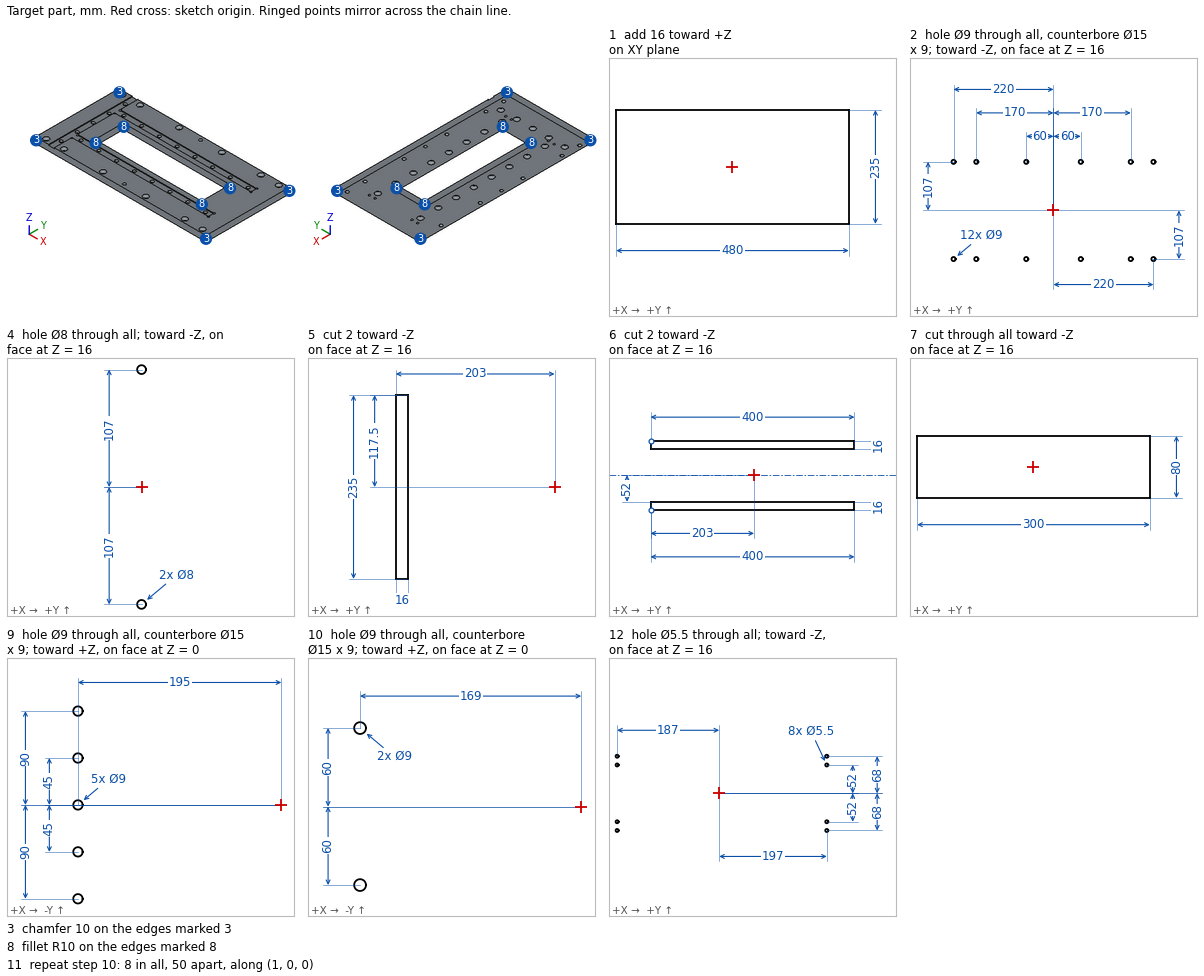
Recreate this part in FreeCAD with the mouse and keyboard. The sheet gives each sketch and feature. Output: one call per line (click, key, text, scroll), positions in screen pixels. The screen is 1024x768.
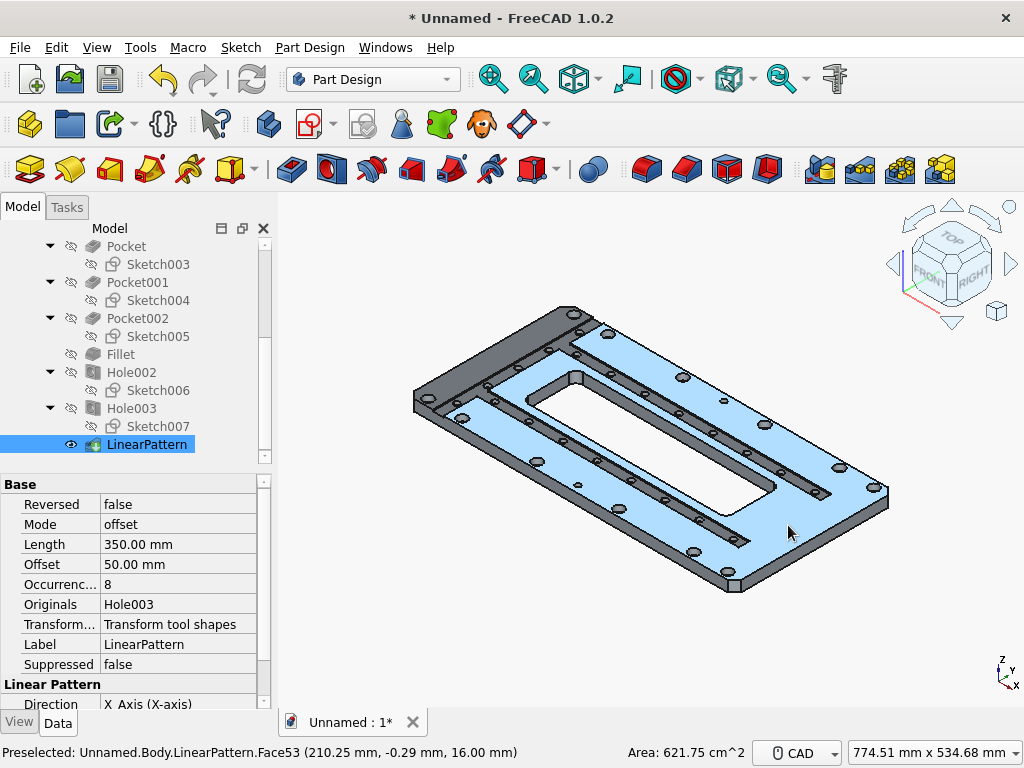
click(310, 124)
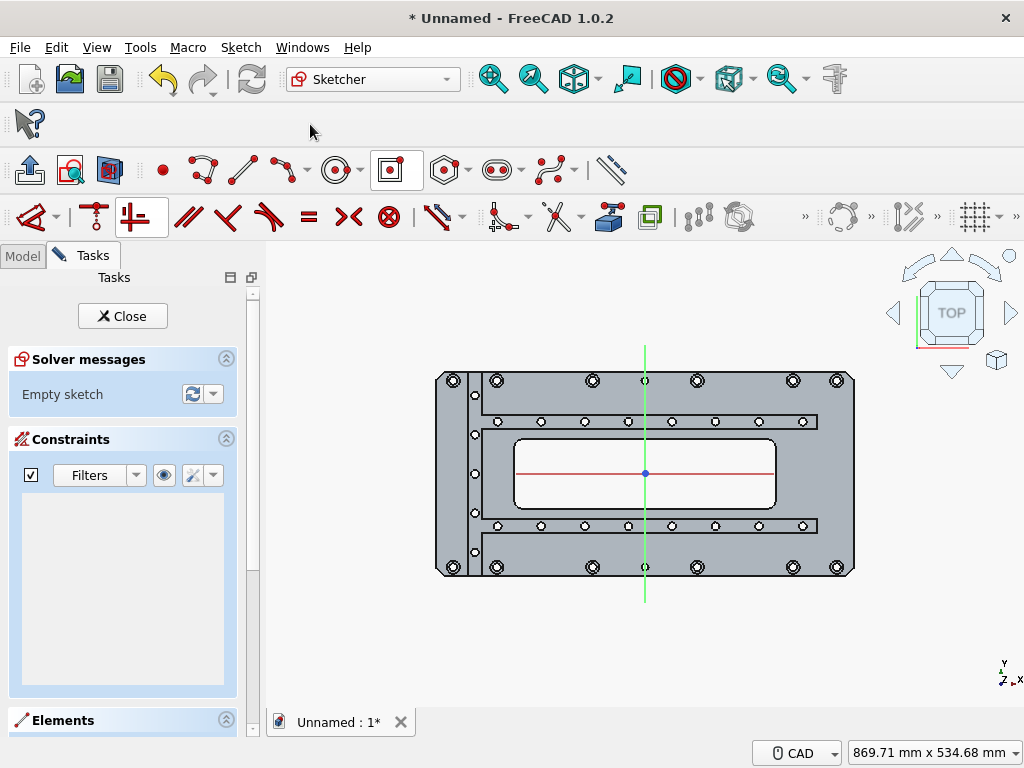
click(336, 170)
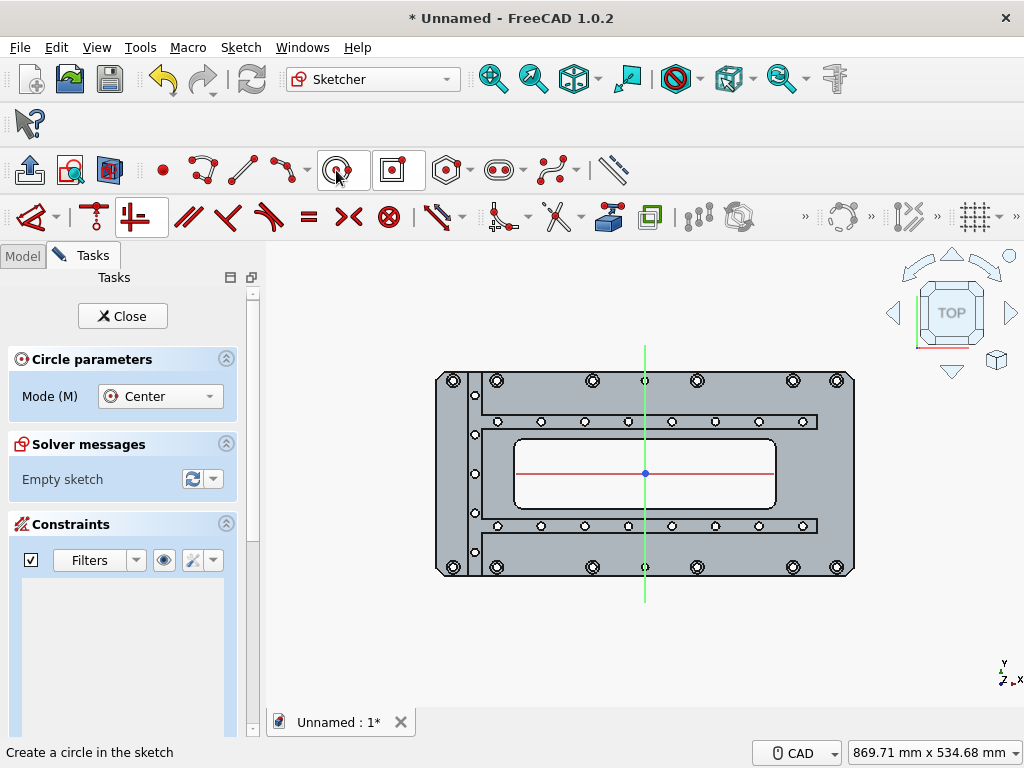
scroll(817, 533, up, 12)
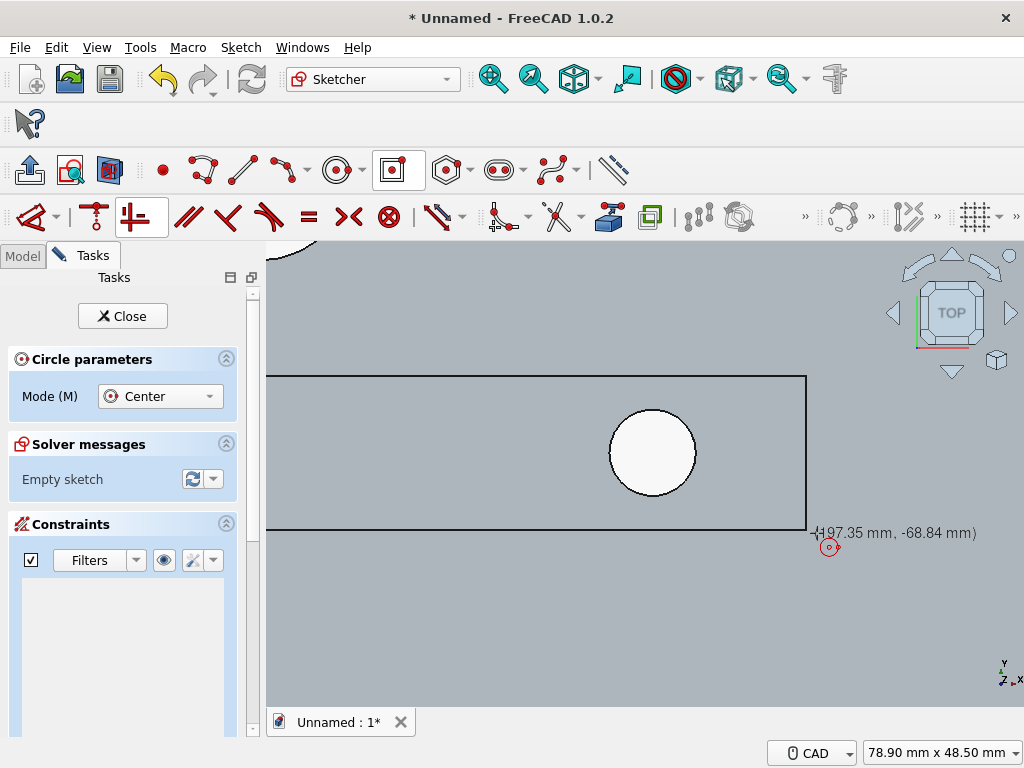
scroll(778, 548, down, 11)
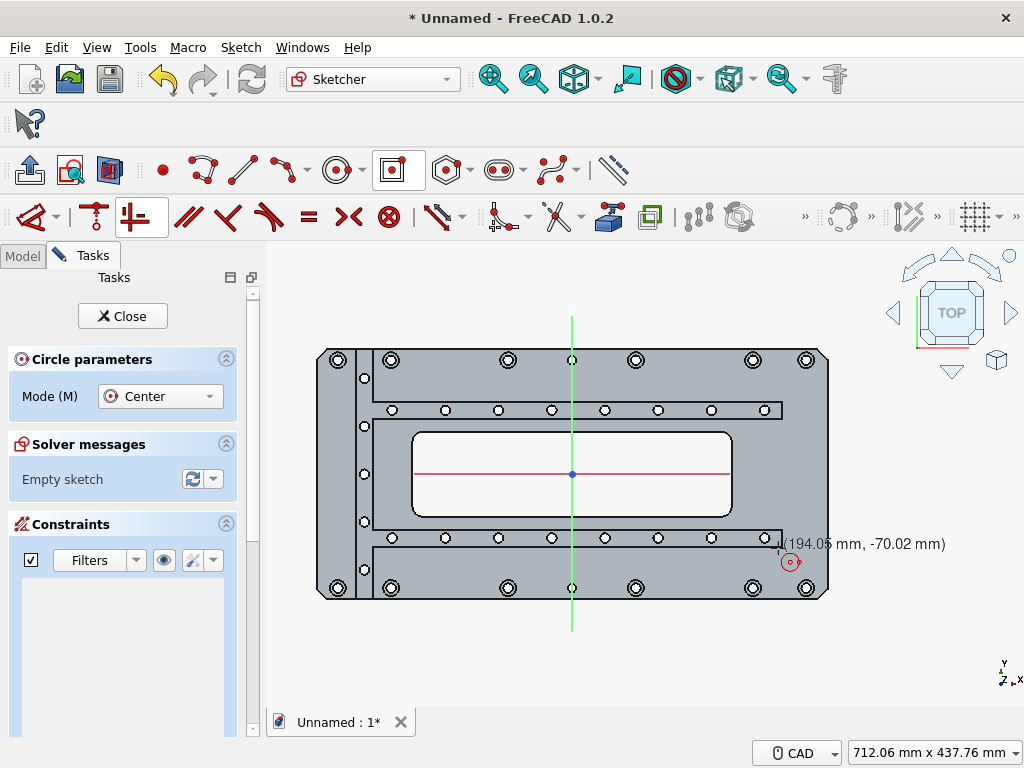
click(782, 547)
move(784, 544)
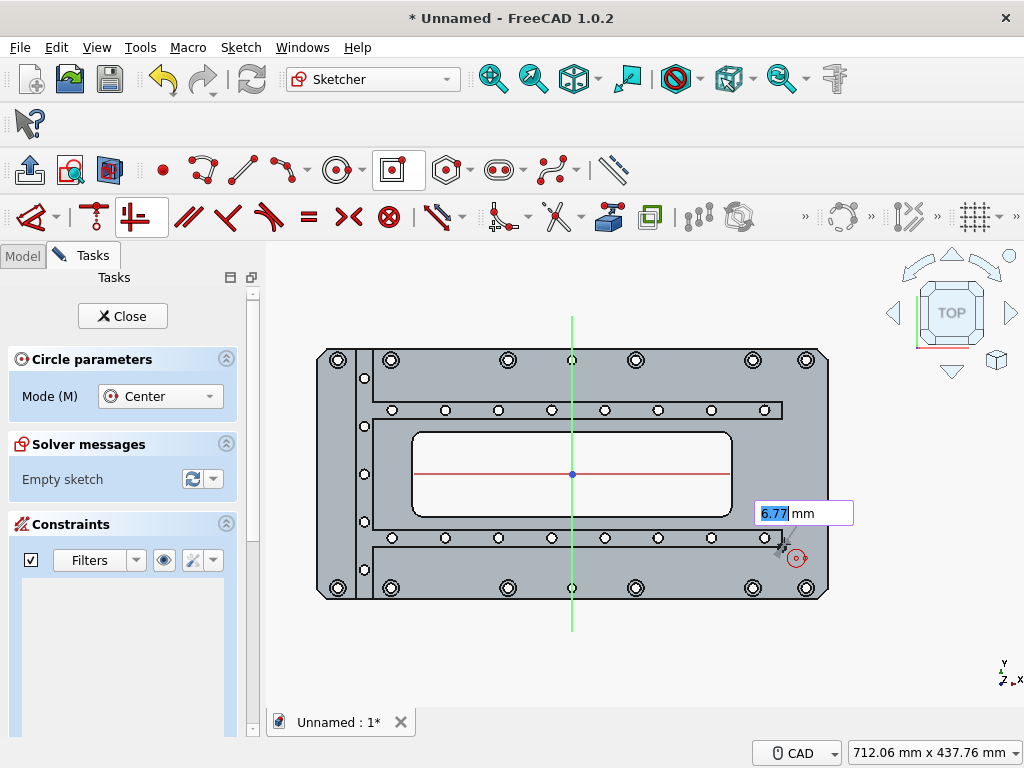
text(5.5)
key(Return)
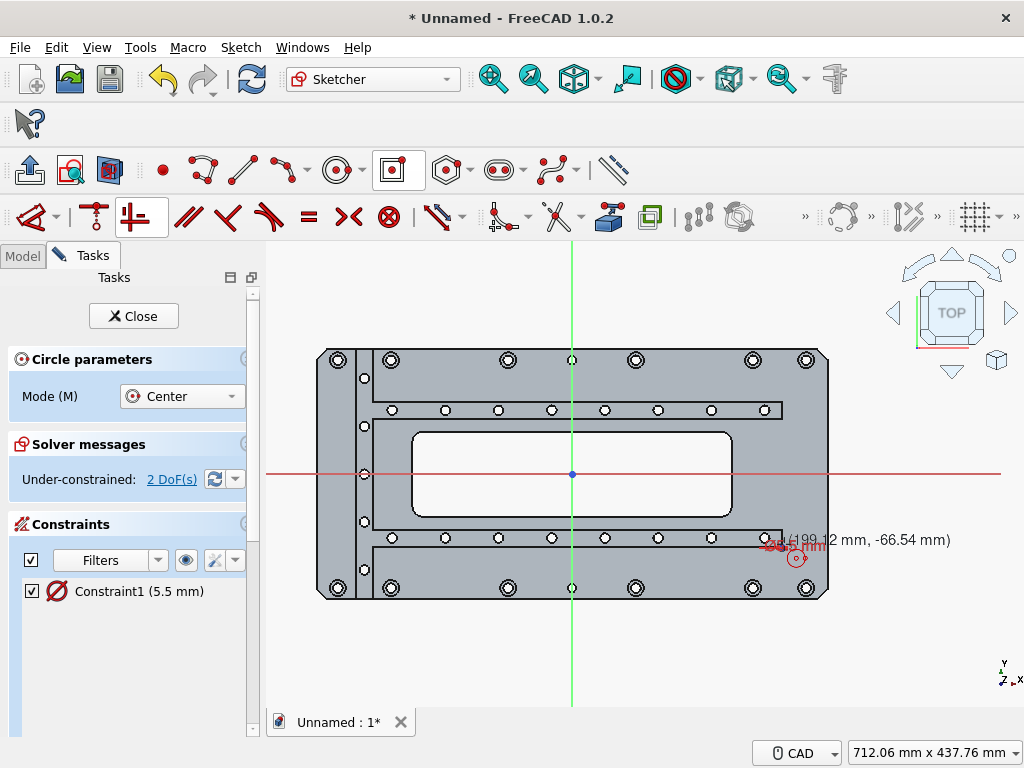
scroll(782, 530, up, 11)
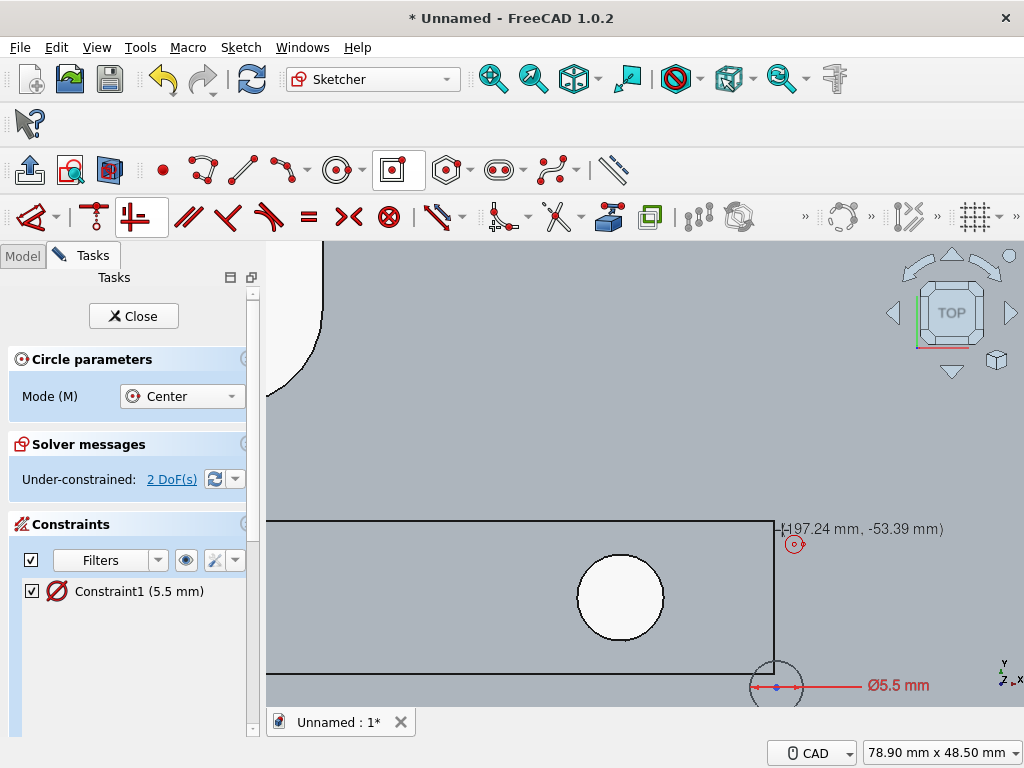
scroll(782, 530, down, 11)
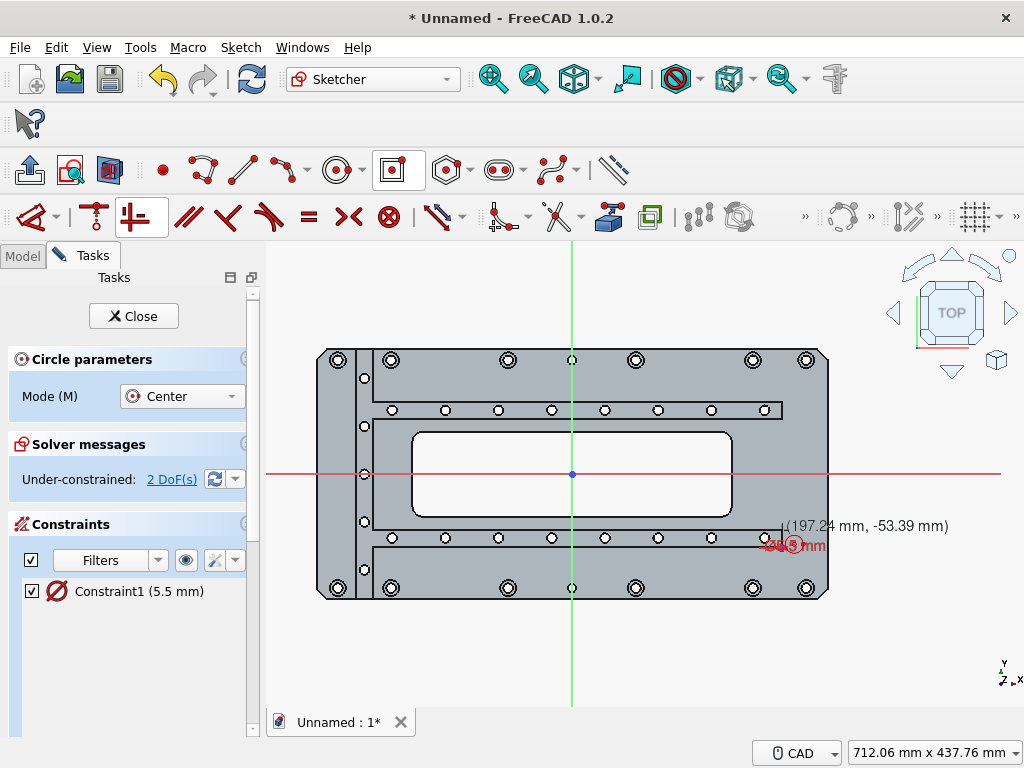
click(782, 530)
move(784, 527)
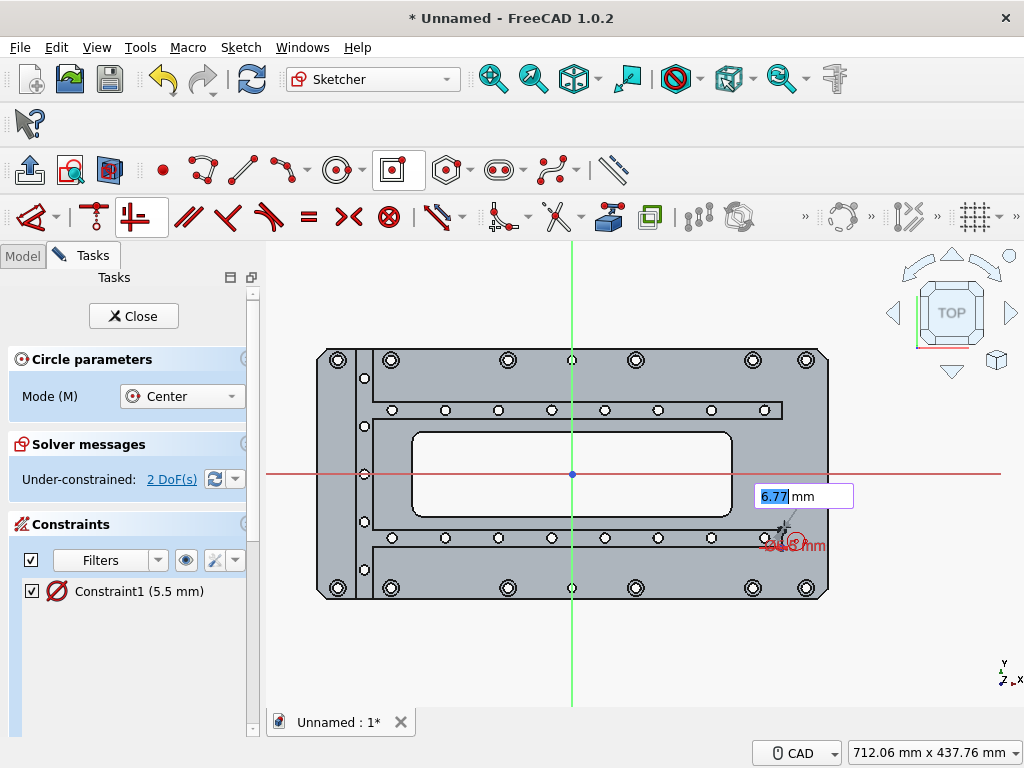
text(5.5)
key(Return)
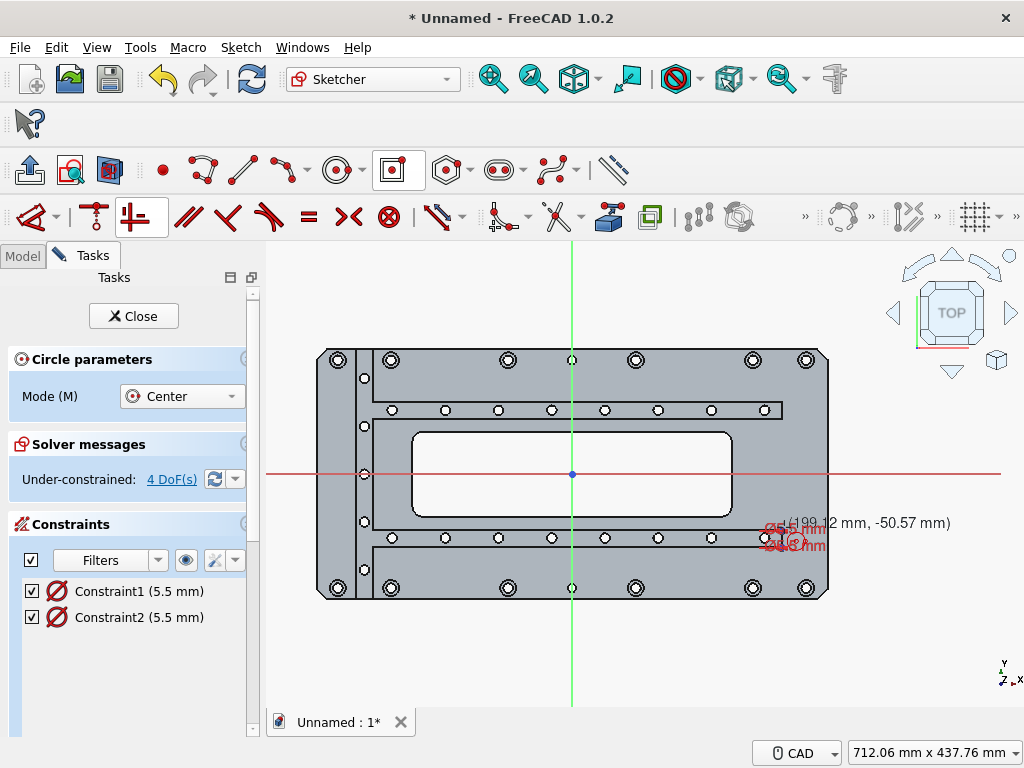
scroll(782, 419, up, 11)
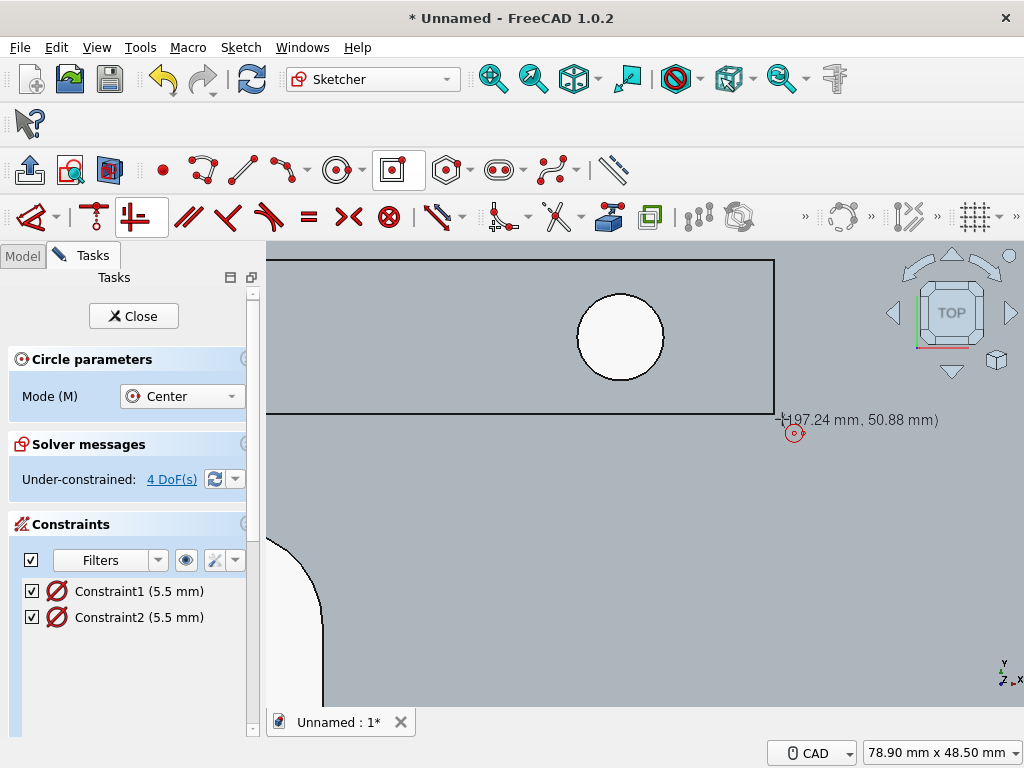
scroll(782, 419, down, 11)